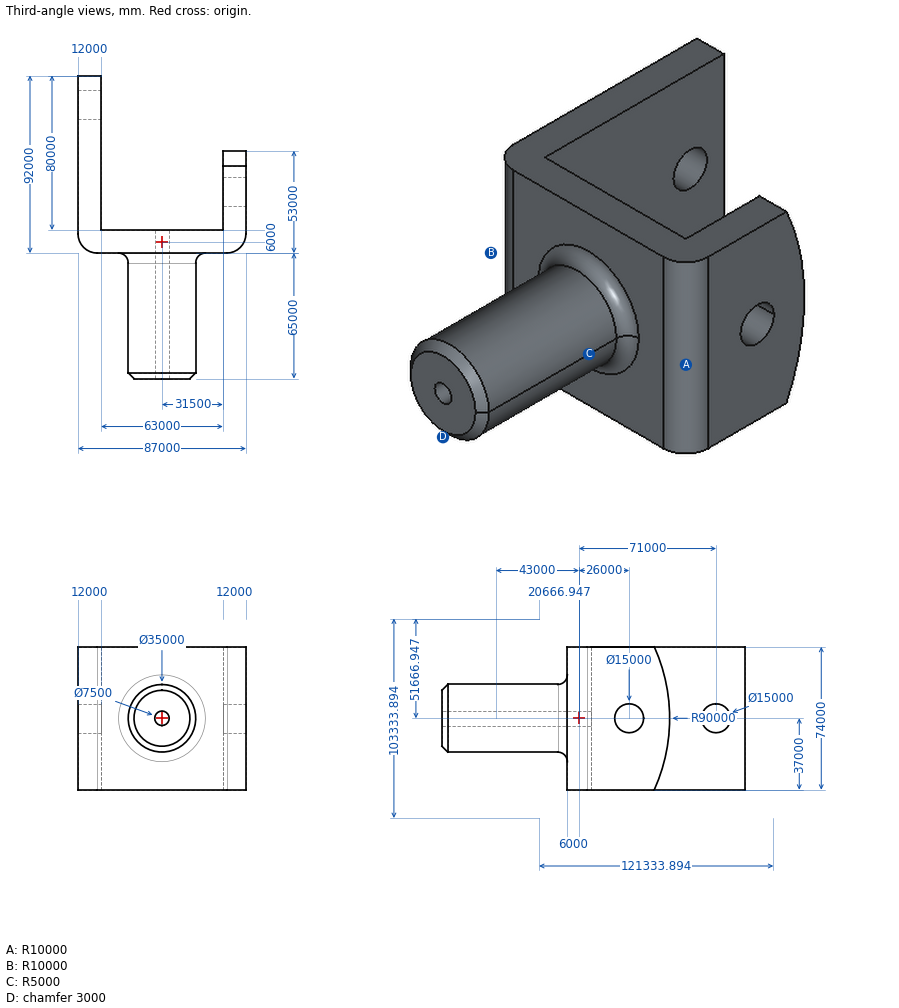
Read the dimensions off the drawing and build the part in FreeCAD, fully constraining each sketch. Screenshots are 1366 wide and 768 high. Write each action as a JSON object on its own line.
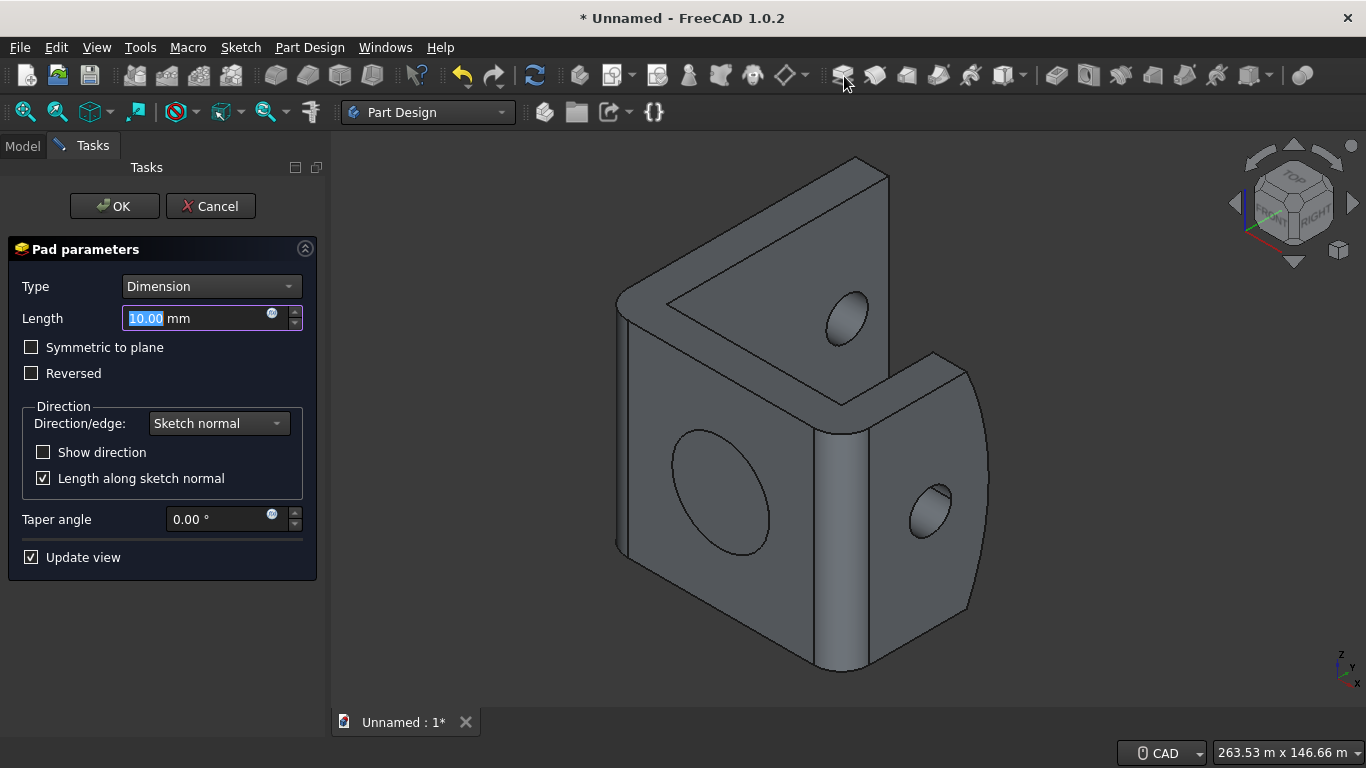
{"action": "type", "text": "65000"}
{"action": "key", "text": "Tab"}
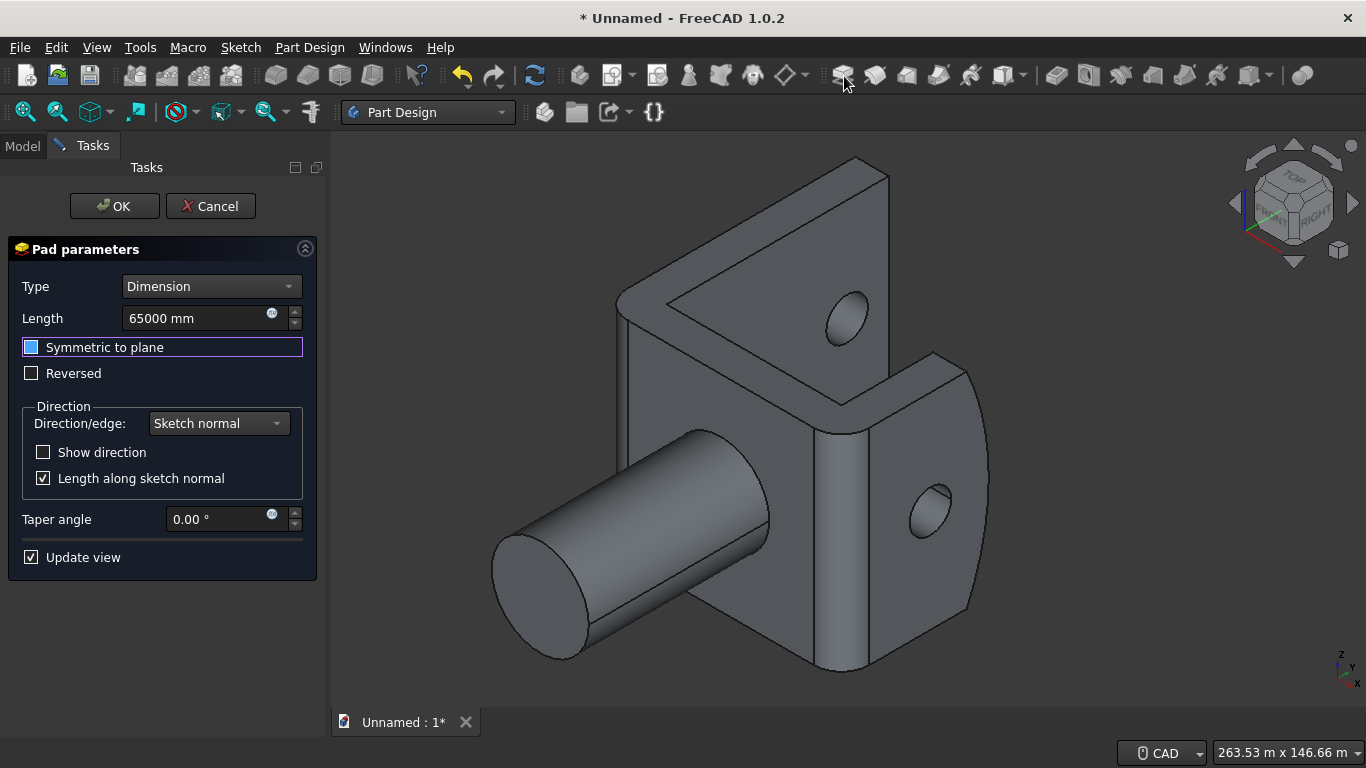
{"action": "left_click", "coordinate": [115, 206]}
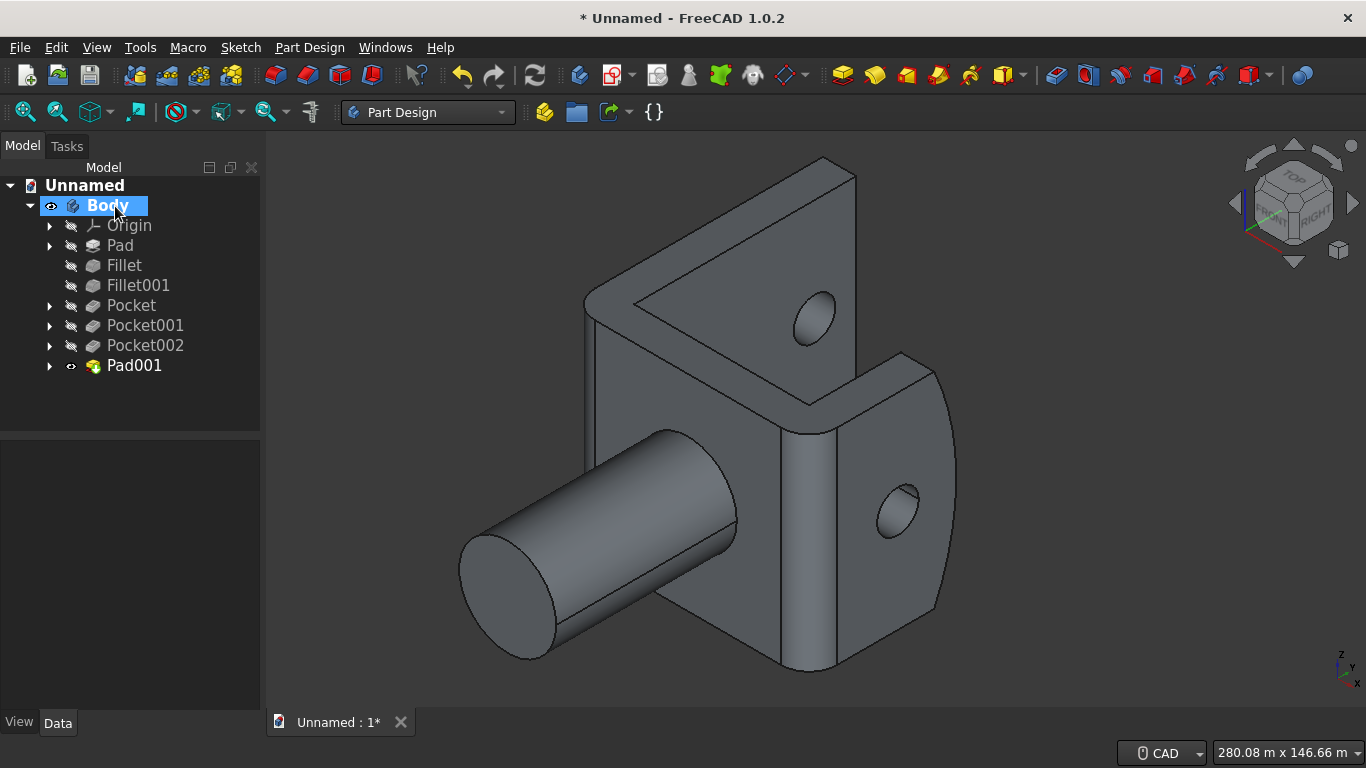
{"action": "left_click", "coordinate": [26, 112]}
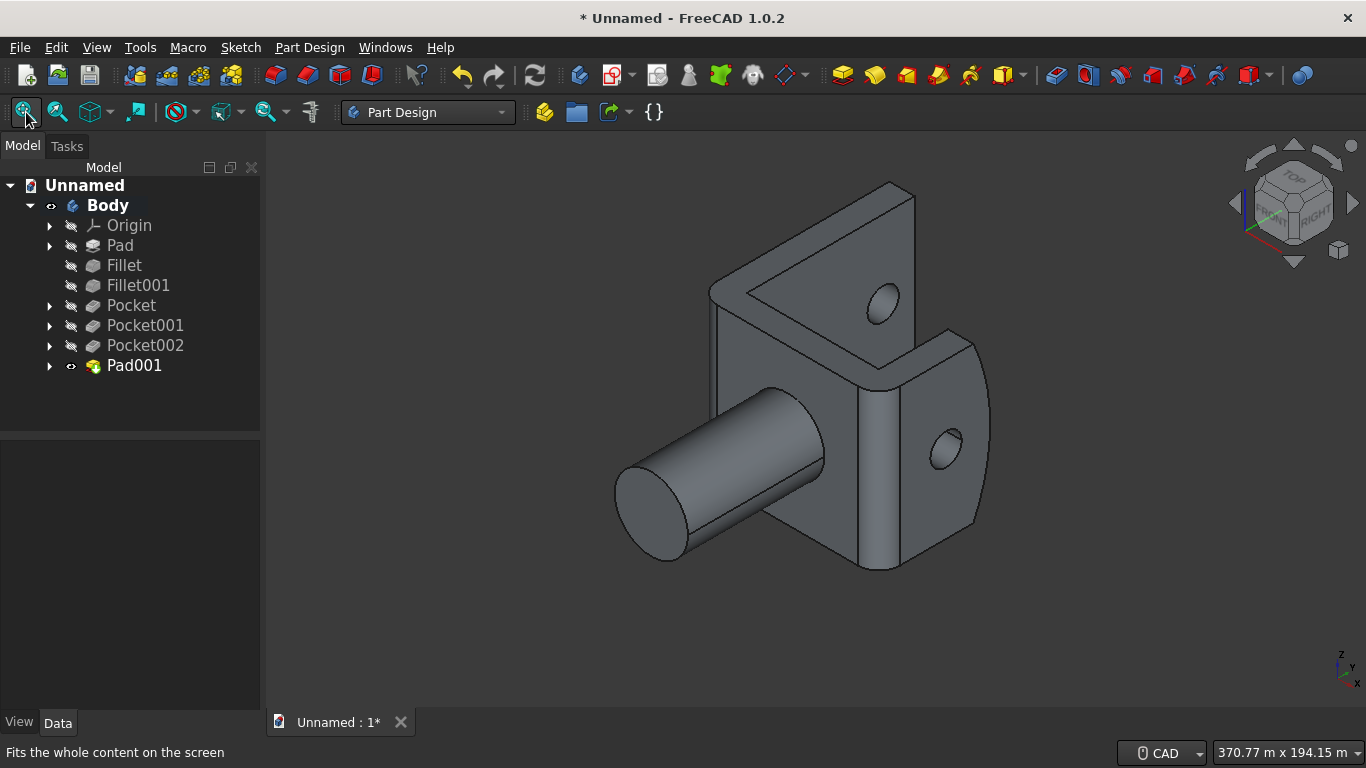
{"action": "key", "text": "2"}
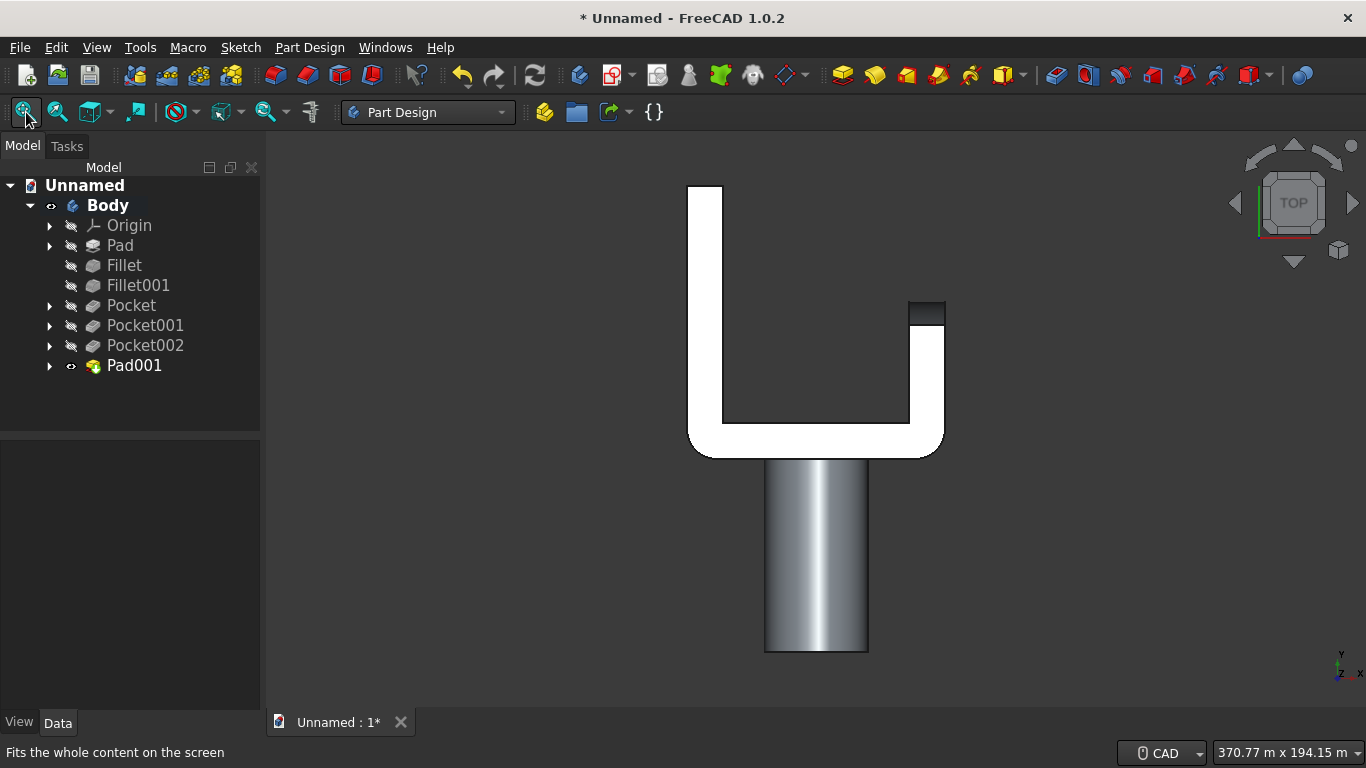
{"action": "key", "text": "0"}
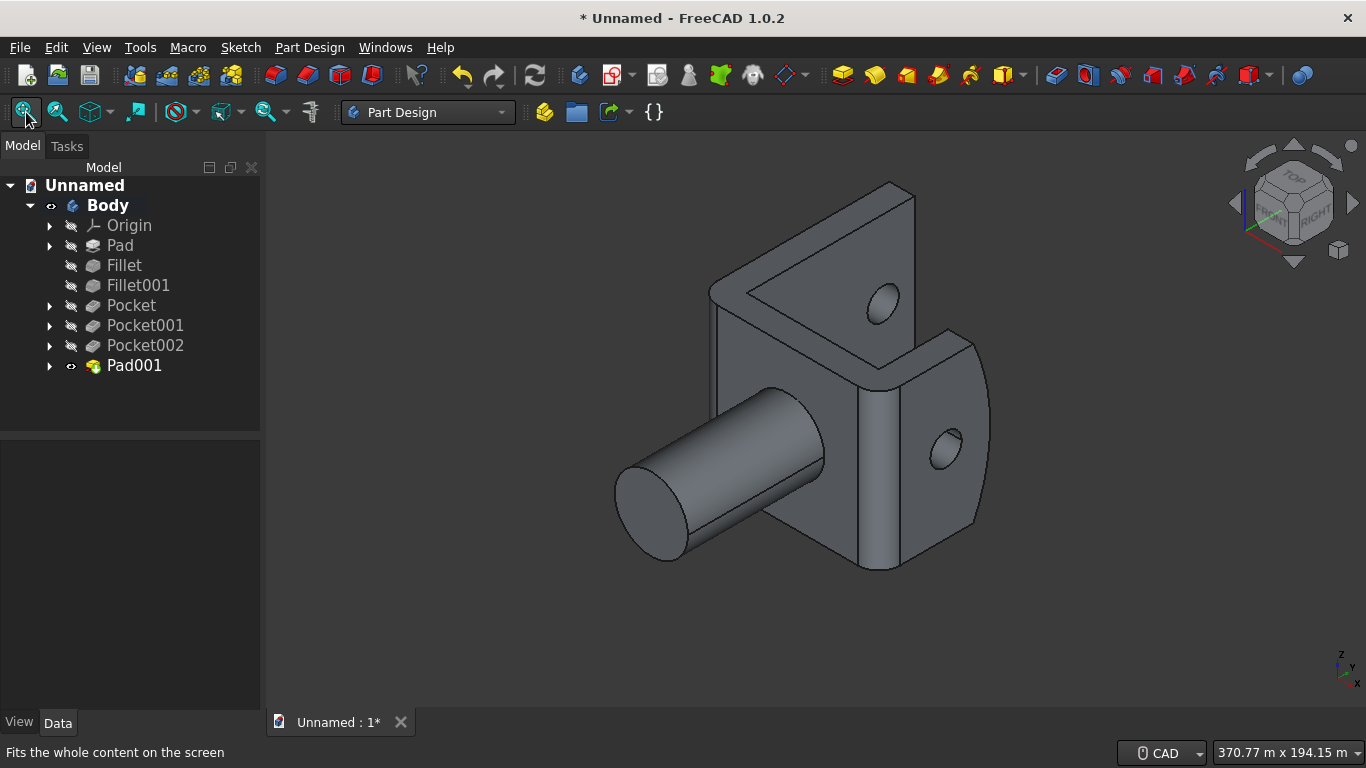
{"action": "key", "text": "1"}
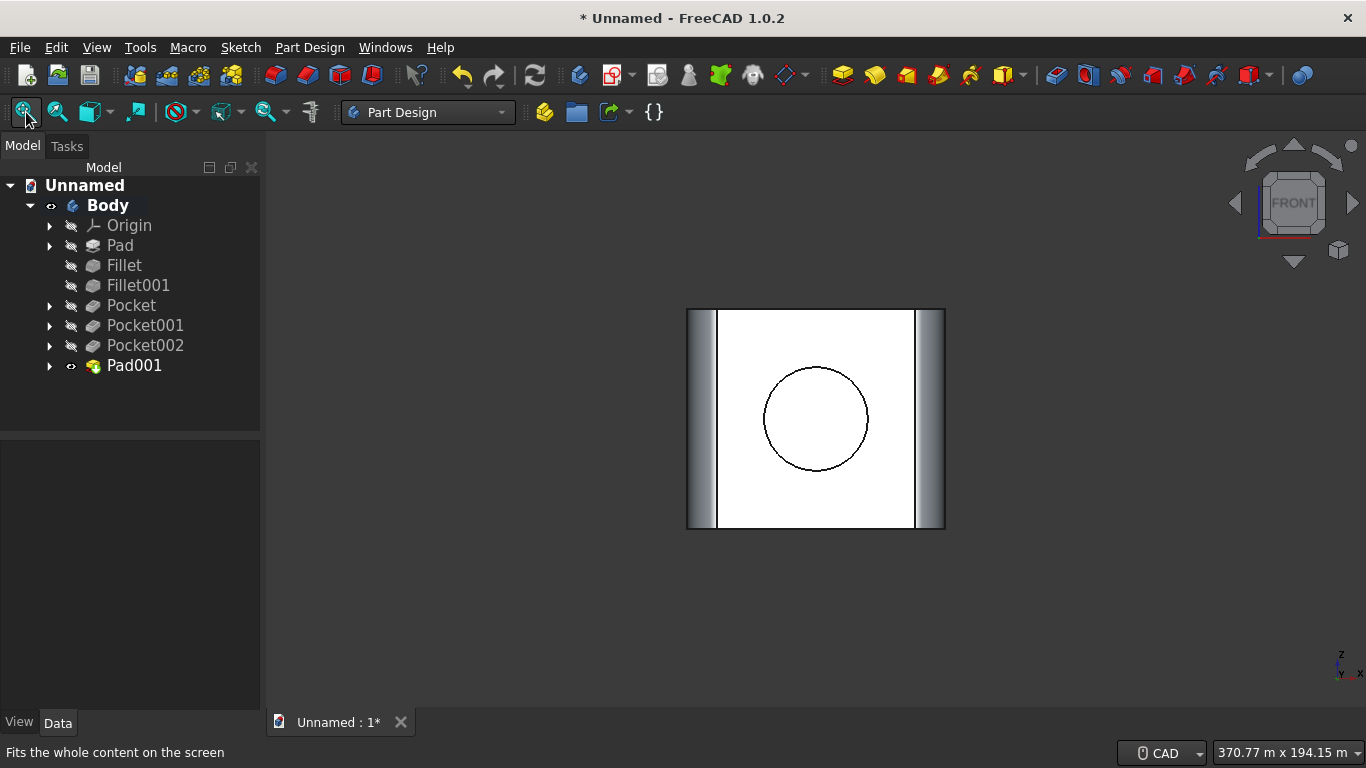
{"action": "left_click", "coordinate": [26, 112]}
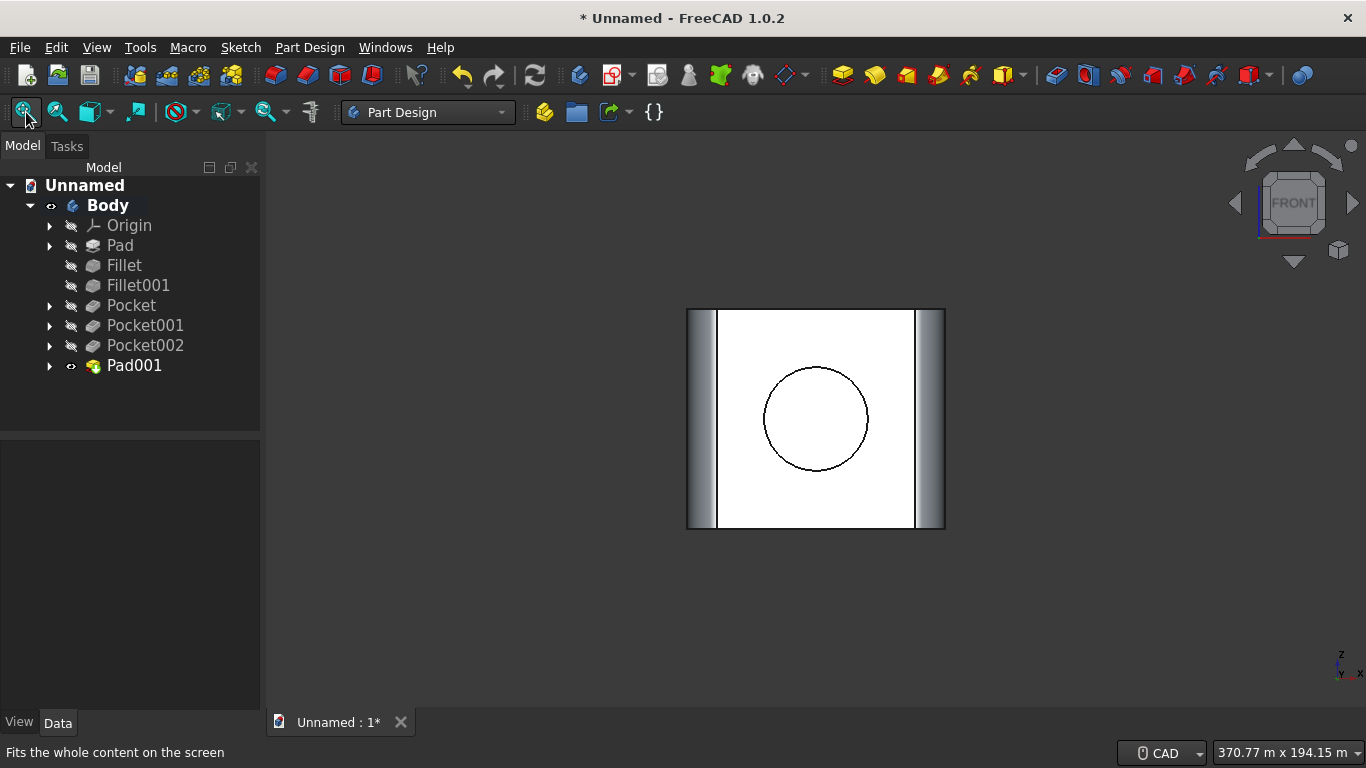
{"action": "key", "text": "3"}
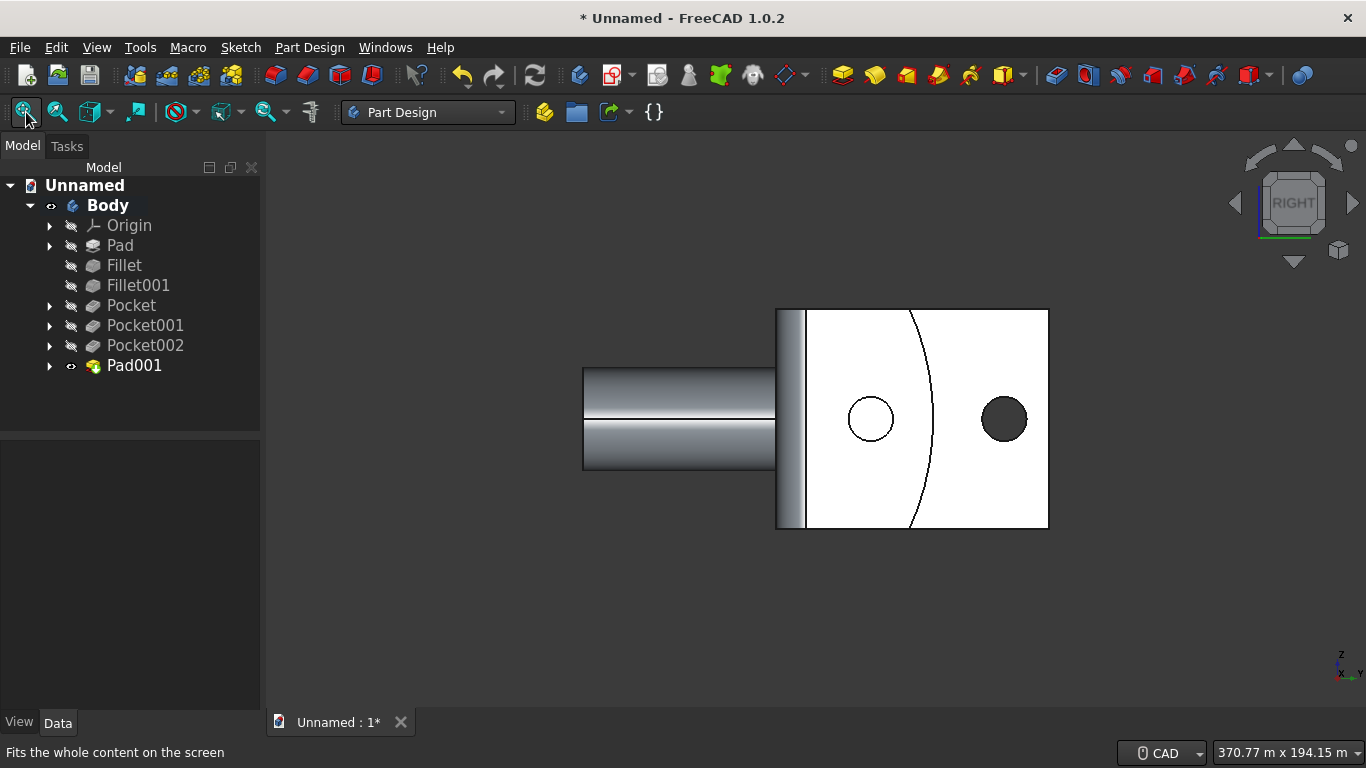
{"action": "left_click", "coordinate": [26, 112]}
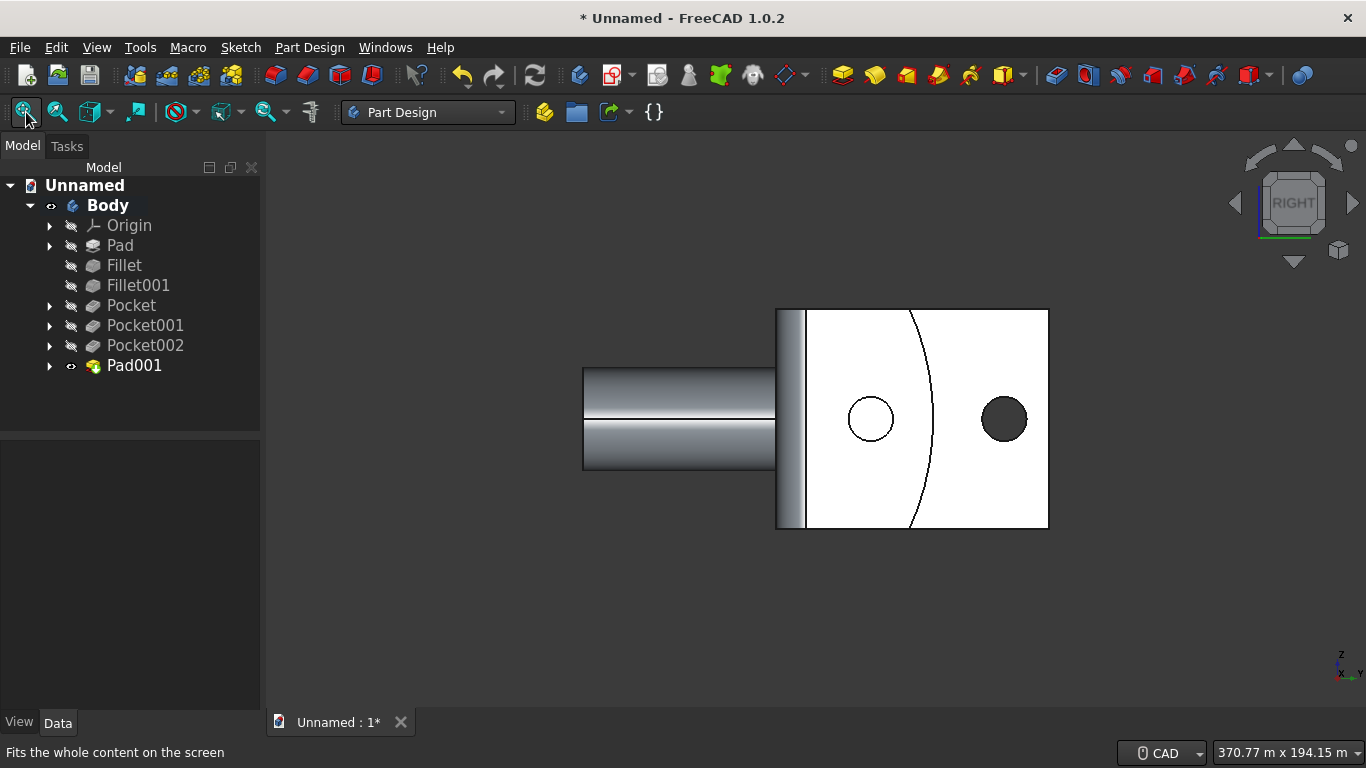
{"action": "key", "text": "5"}